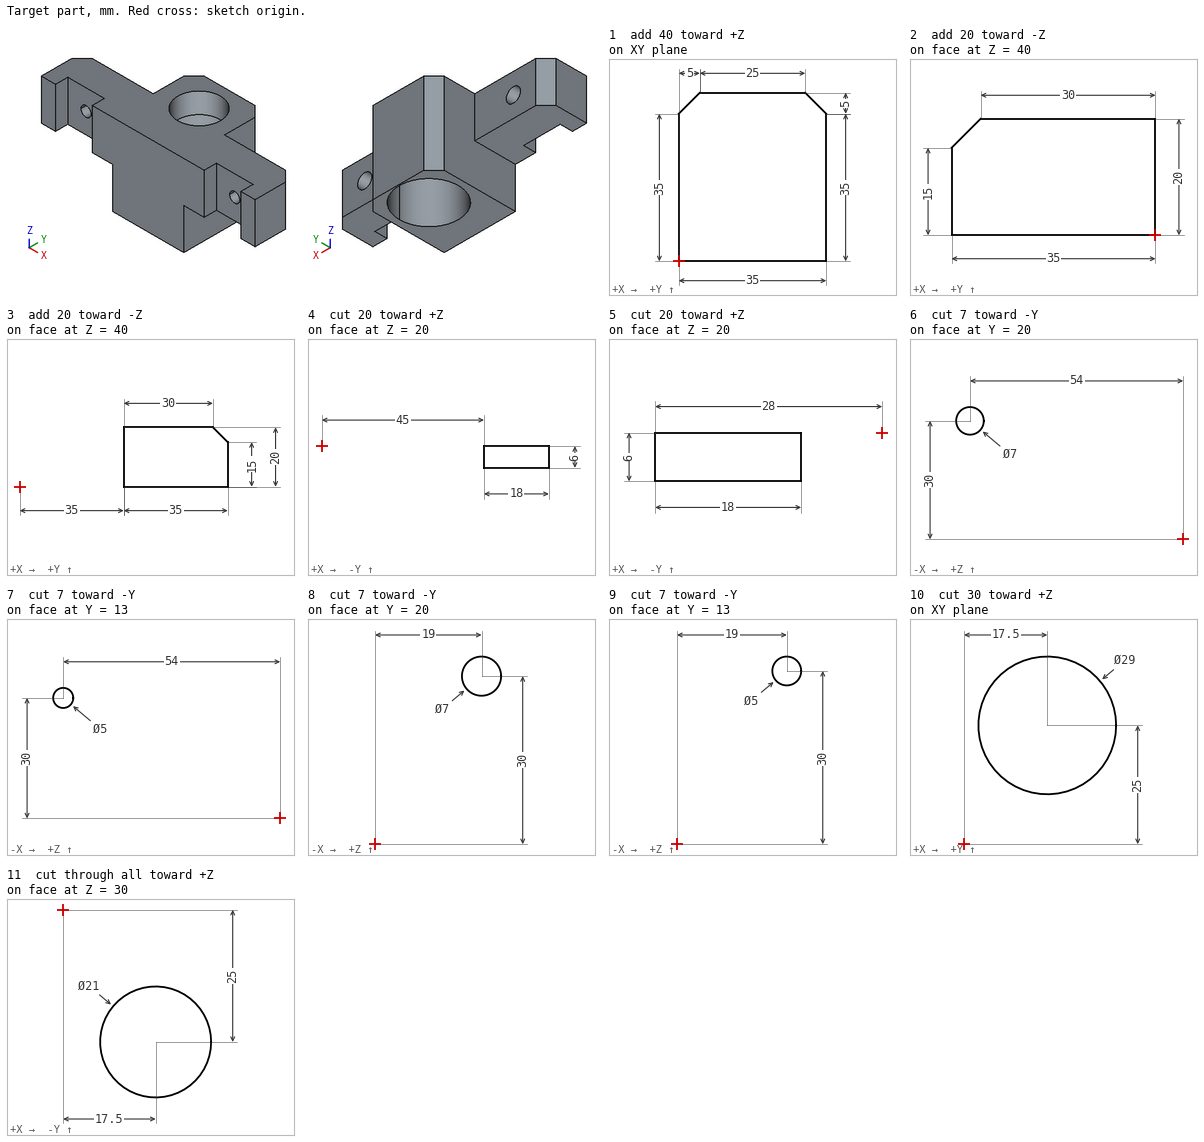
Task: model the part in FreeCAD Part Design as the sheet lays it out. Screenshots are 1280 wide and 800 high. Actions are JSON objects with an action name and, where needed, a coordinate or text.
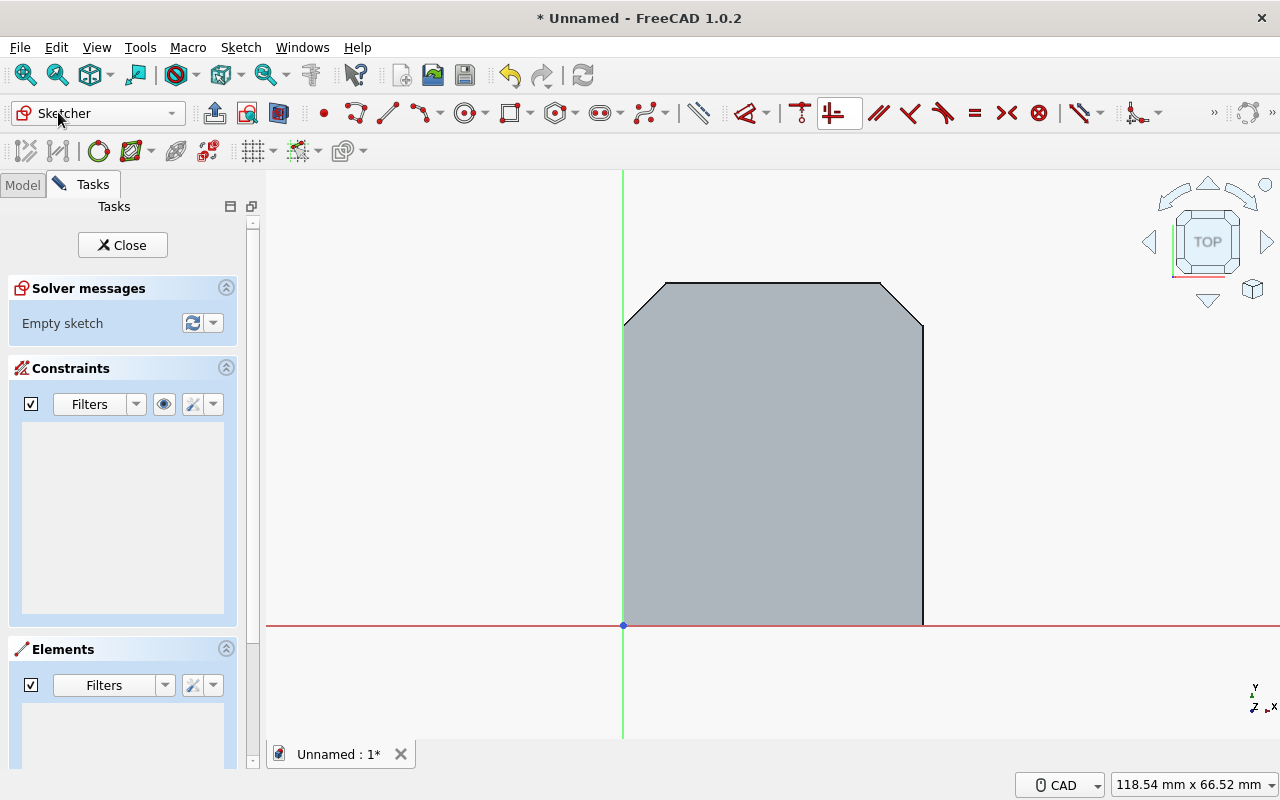
{"action": "scroll", "coordinate": [294, 644], "scroll_direction": "up", "scroll_amount": 3}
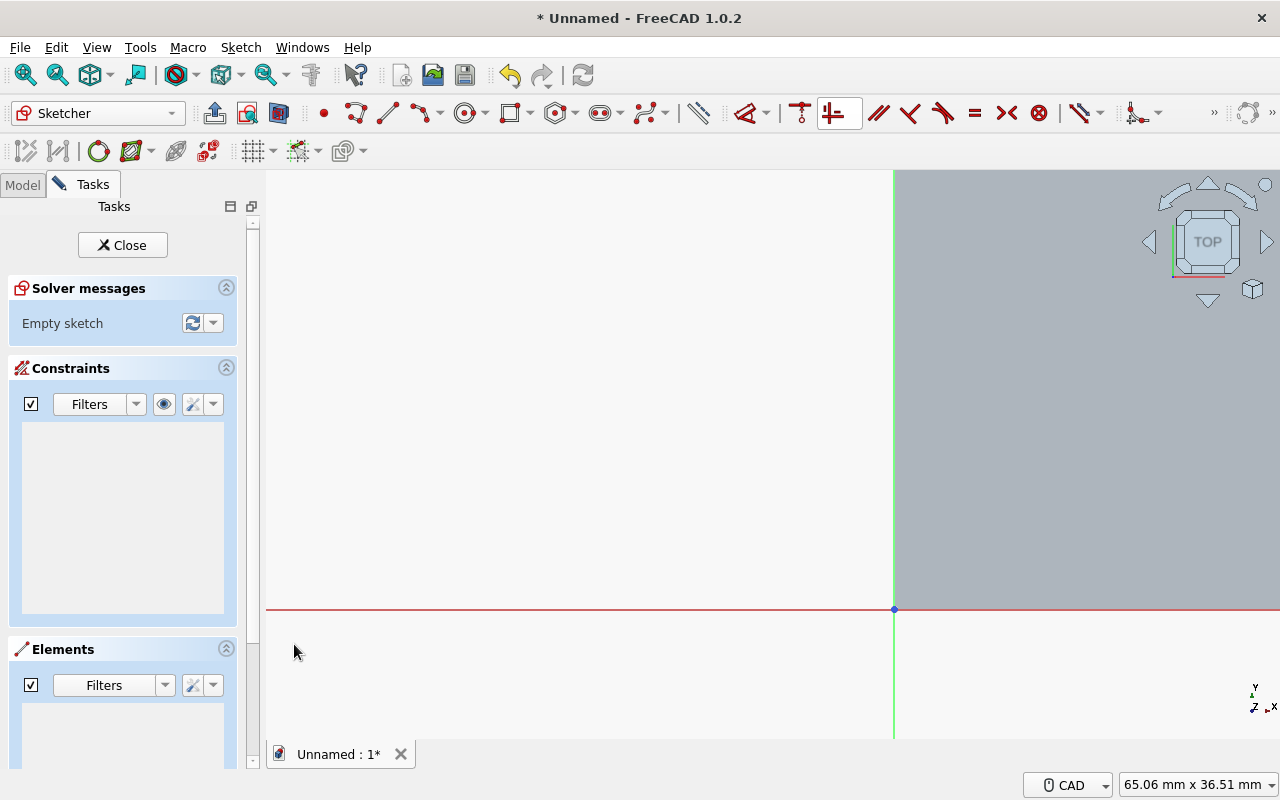
{"action": "left_click", "coordinate": [356, 114]}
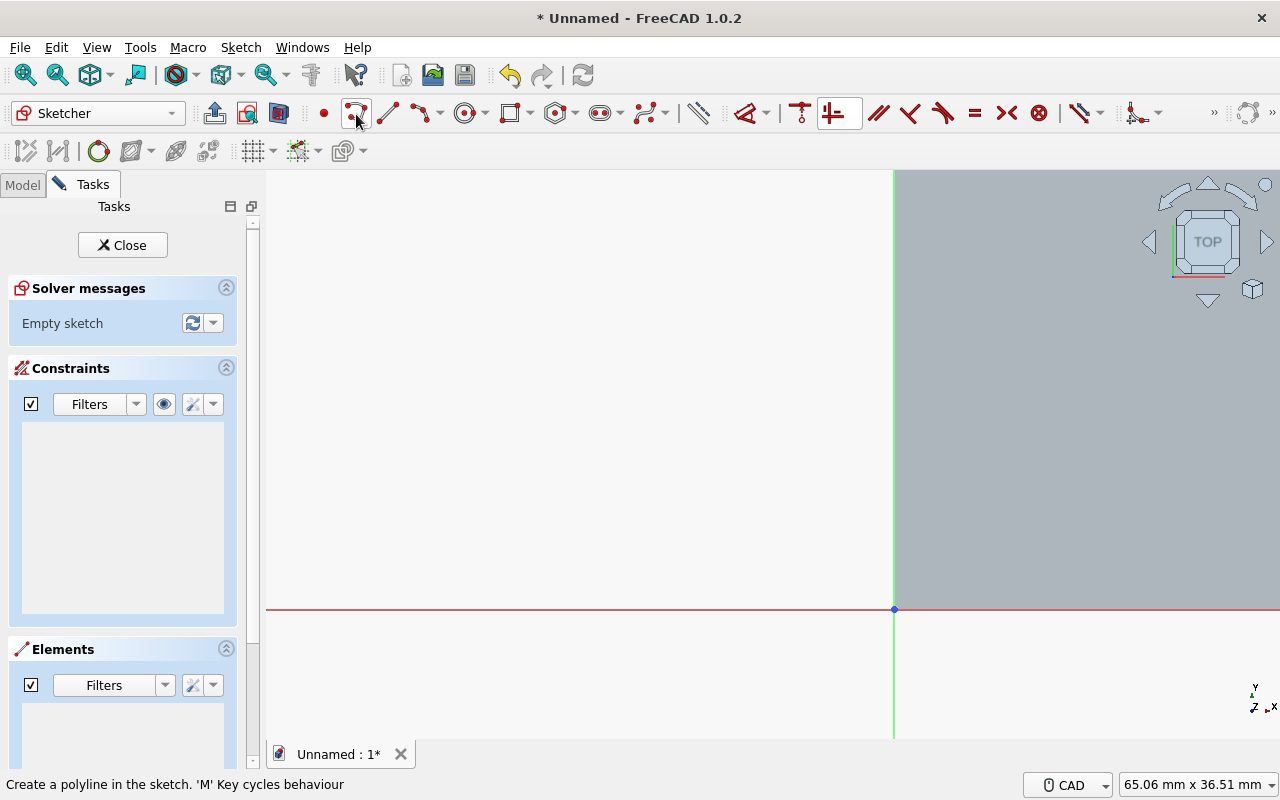
{"action": "left_click", "coordinate": [894, 610]}
{"action": "left_click", "coordinate": [885, 298]}
{"action": "left_click", "coordinate": [426, 298]}
{"action": "left_click", "coordinate": [349, 376]}
{"action": "left_click", "coordinate": [349, 601]}
{"action": "left_click", "coordinate": [894, 610]}
{"action": "key", "text": "Escape"}
{"action": "key", "text": "Escape"}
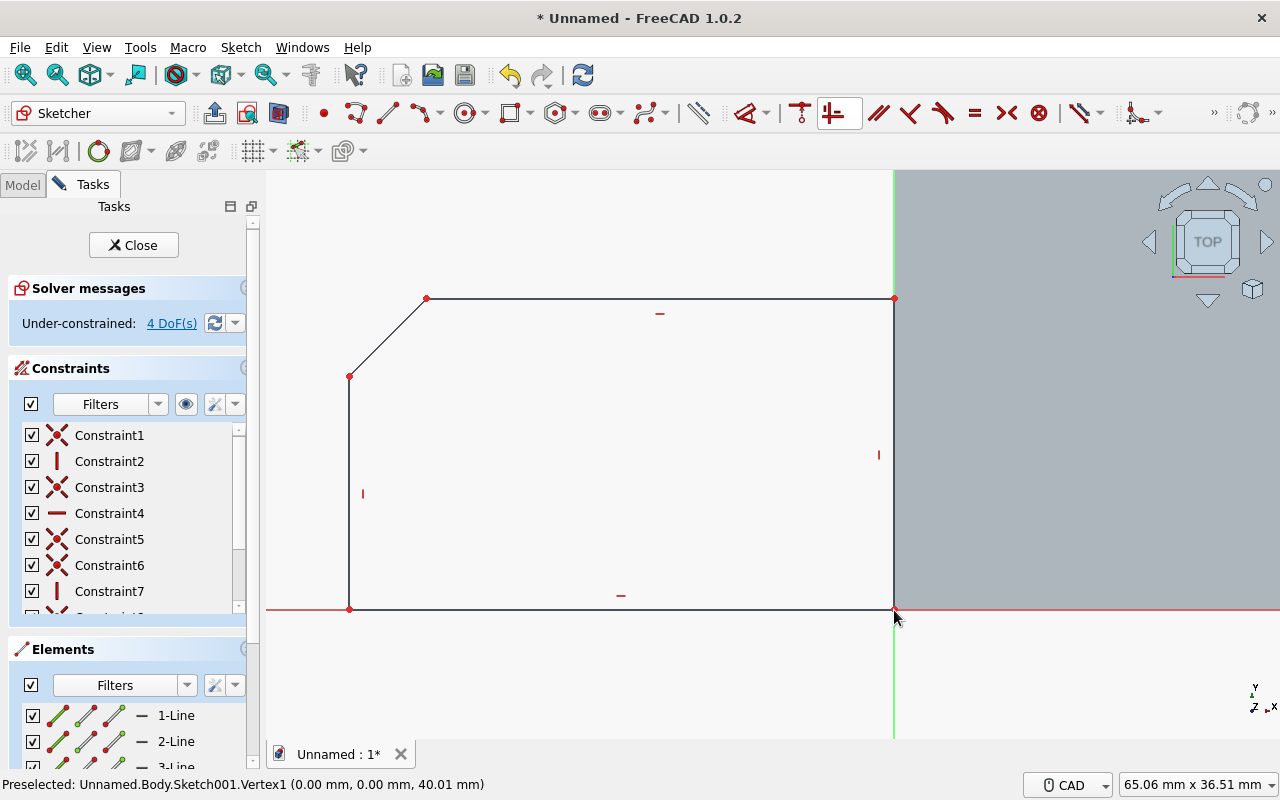
{"action": "left_click", "coordinate": [746, 114]}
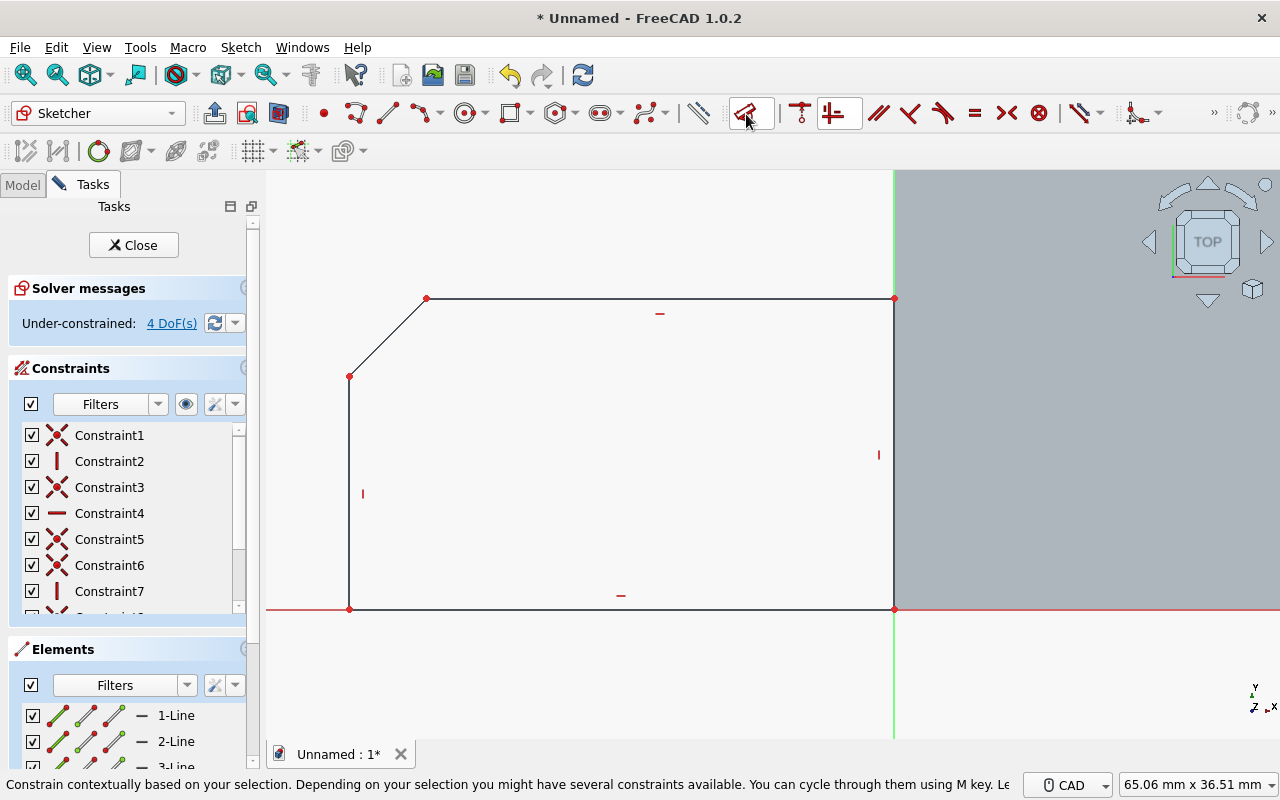
{"action": "left_click", "coordinate": [894, 517]}
{"action": "left_click", "coordinate": [928, 454]}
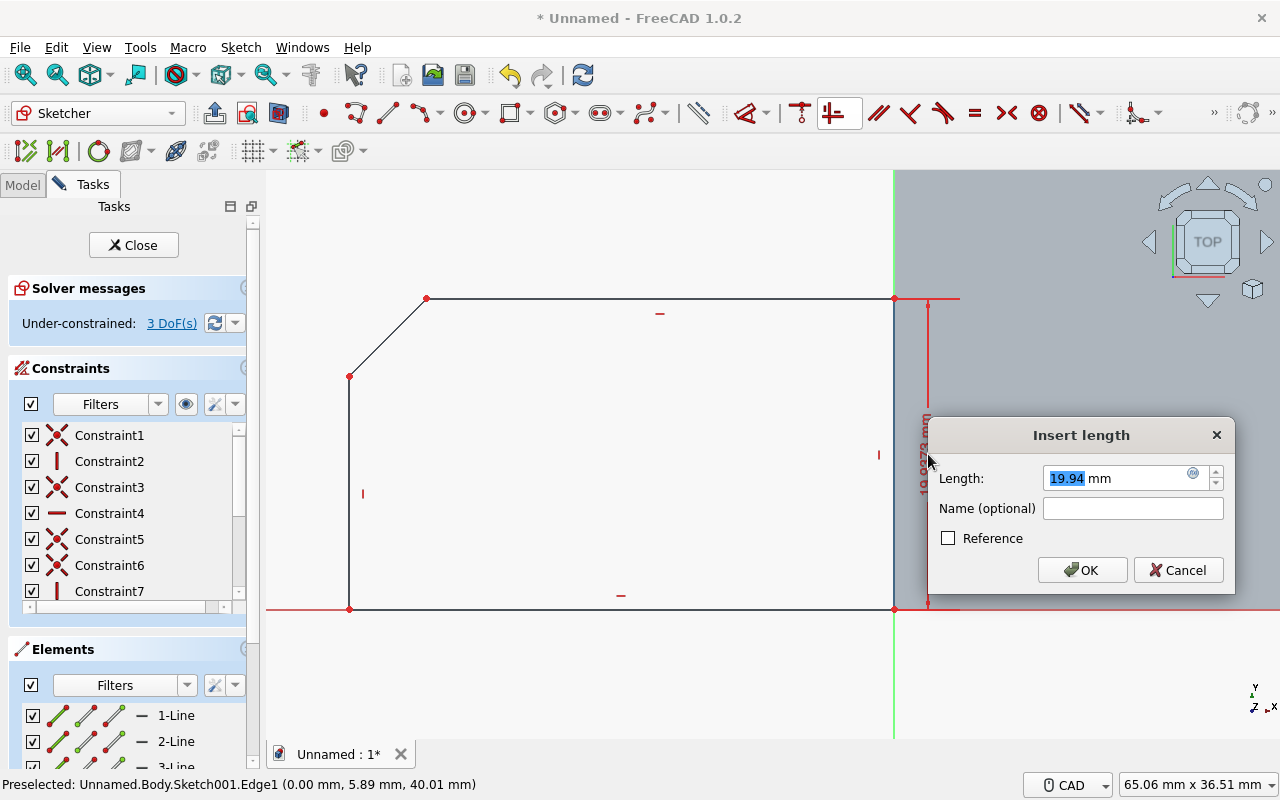
{"action": "type", "text": "20"}
{"action": "key", "text": "Return"}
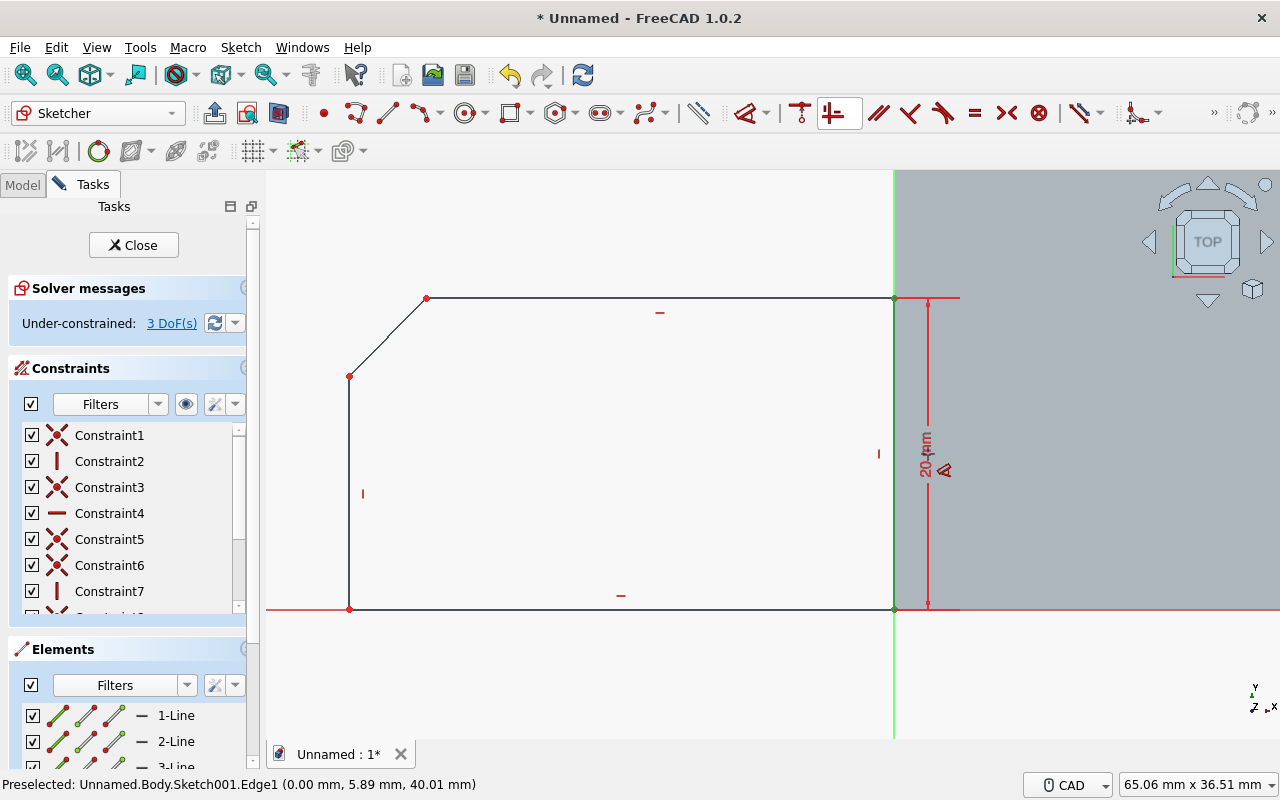
{"action": "left_click", "coordinate": [754, 298]}
{"action": "left_click", "coordinate": [660, 264]}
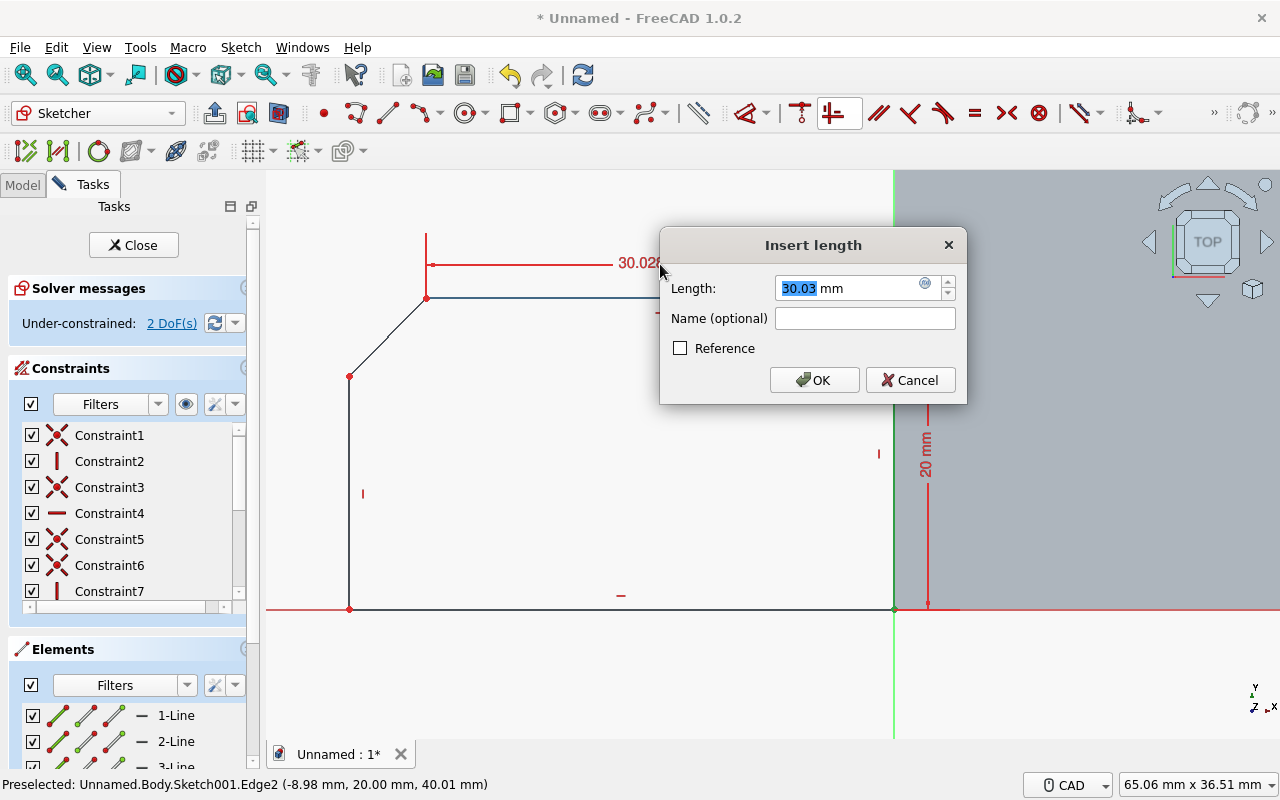
{"action": "type", "text": "30"}
{"action": "key", "text": "Return"}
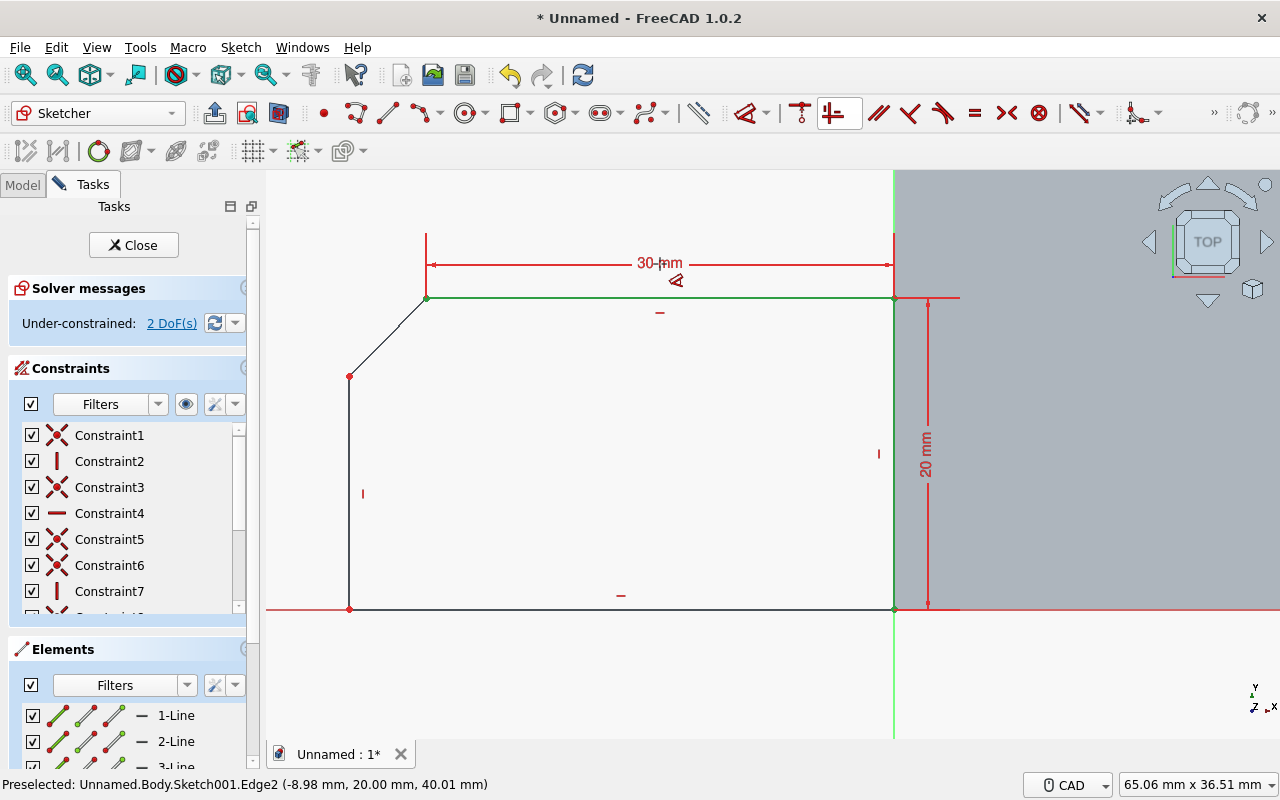
{"action": "left_click", "coordinate": [349, 447]}
{"action": "left_click", "coordinate": [315, 493]}